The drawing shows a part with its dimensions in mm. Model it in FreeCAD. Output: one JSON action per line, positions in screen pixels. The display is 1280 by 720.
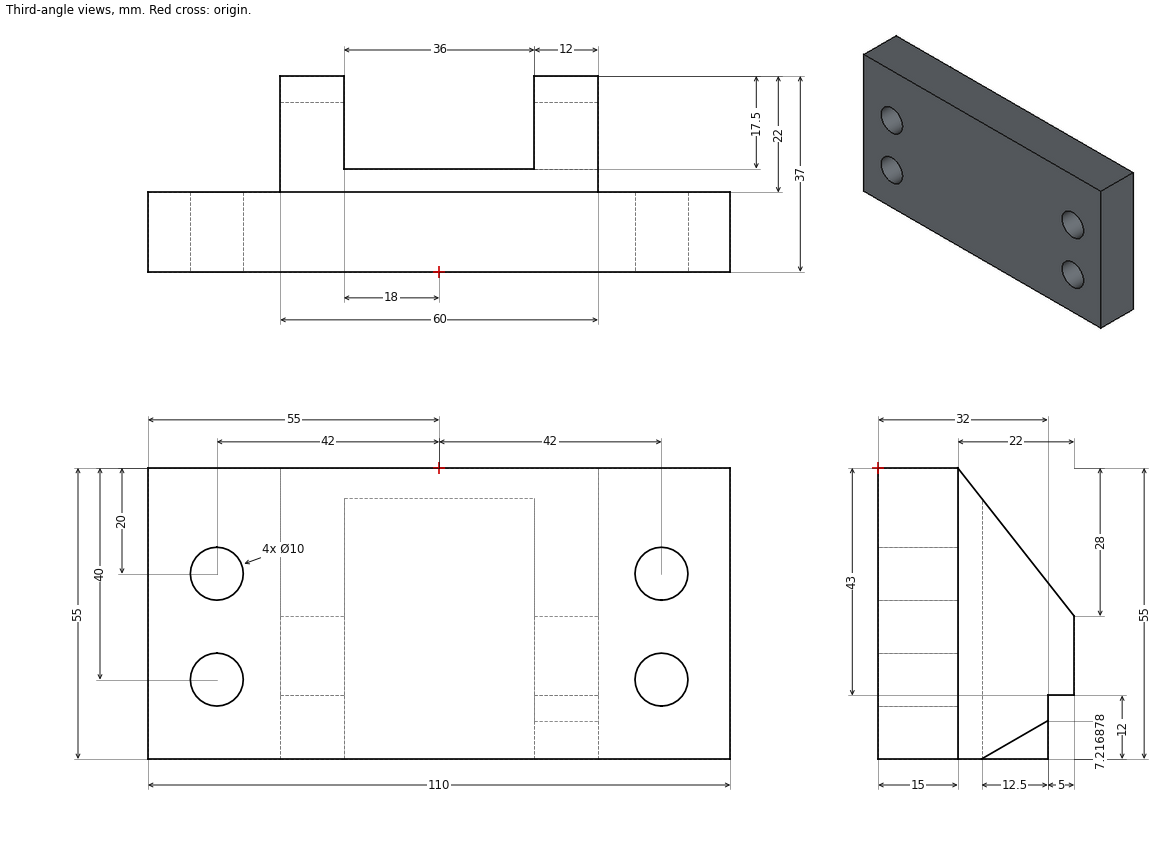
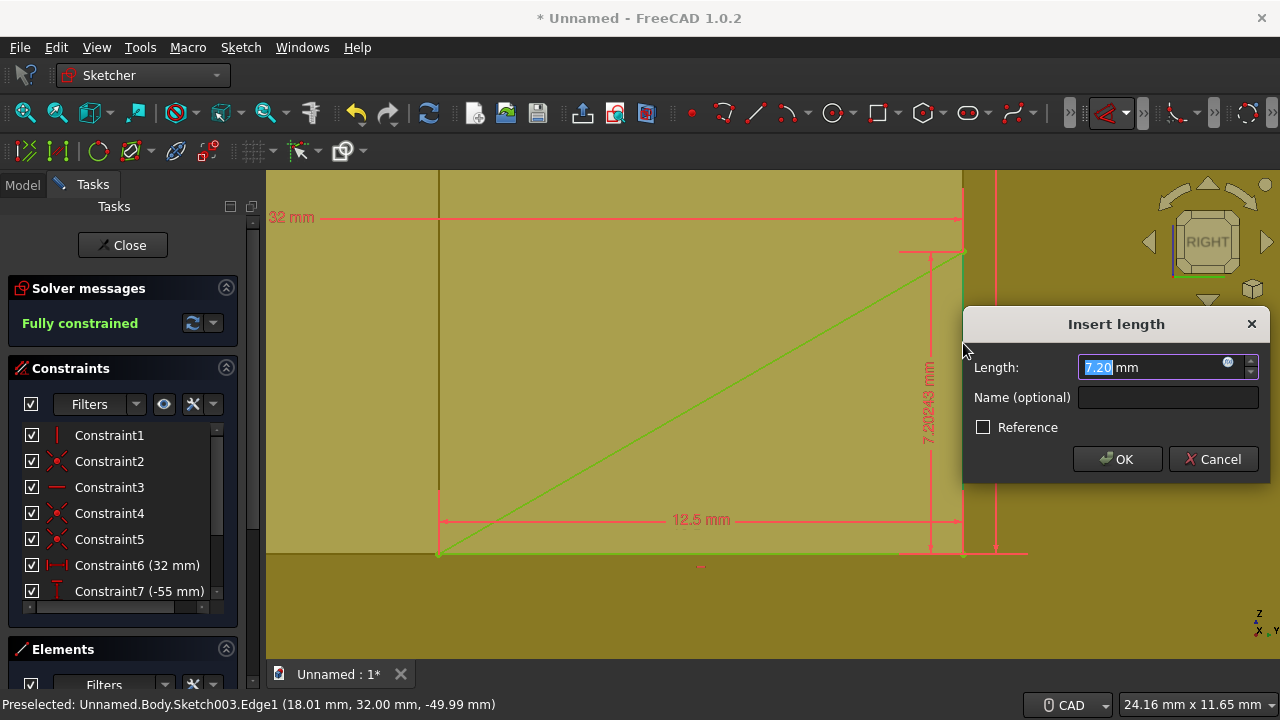
{"action": "type", "text": "7.216878"}
{"action": "key", "text": "Return"}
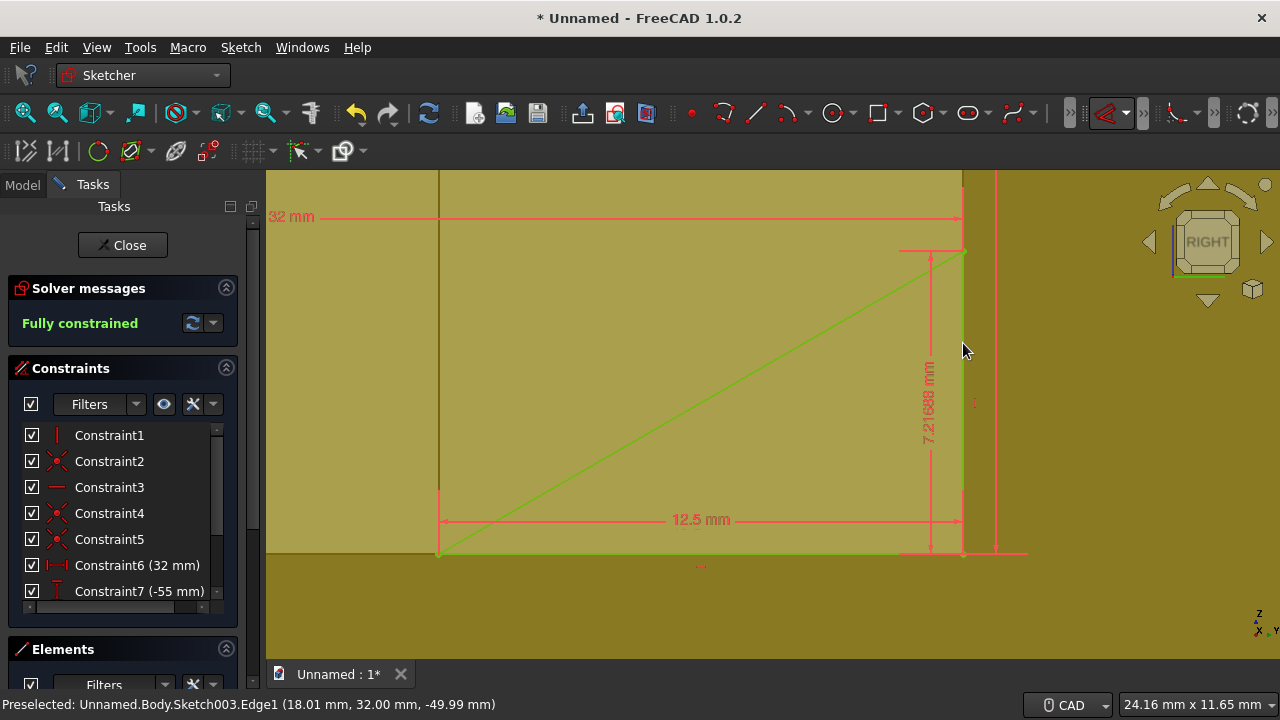
{"action": "left_click", "coordinate": [123, 245]}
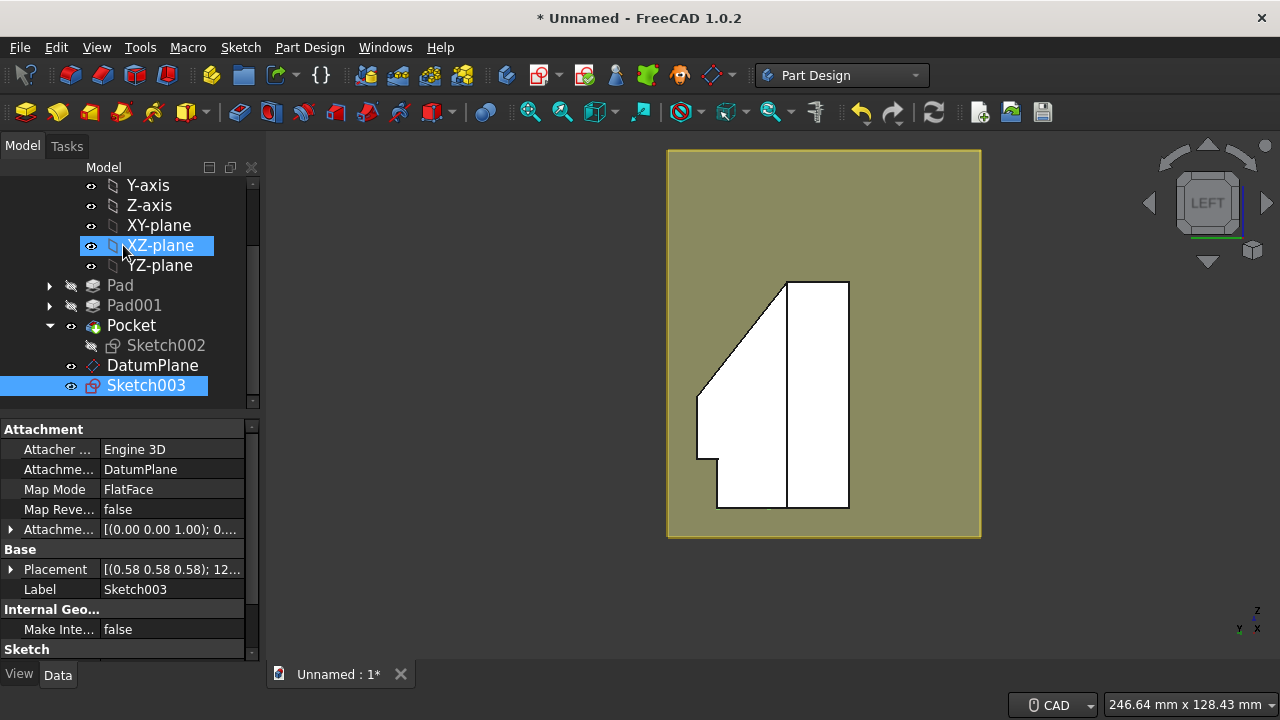
{"action": "left_click", "coordinate": [240, 112]}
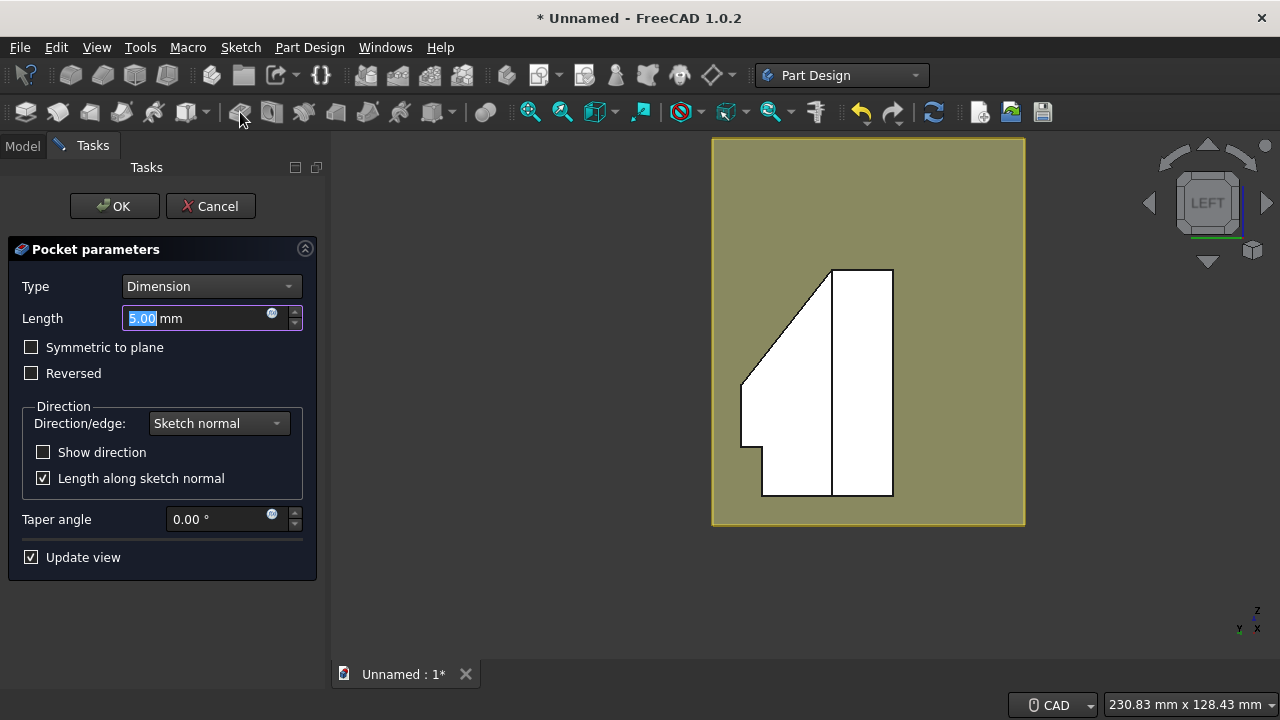
{"action": "type", "text": "12"}
{"action": "key", "text": "Tab"}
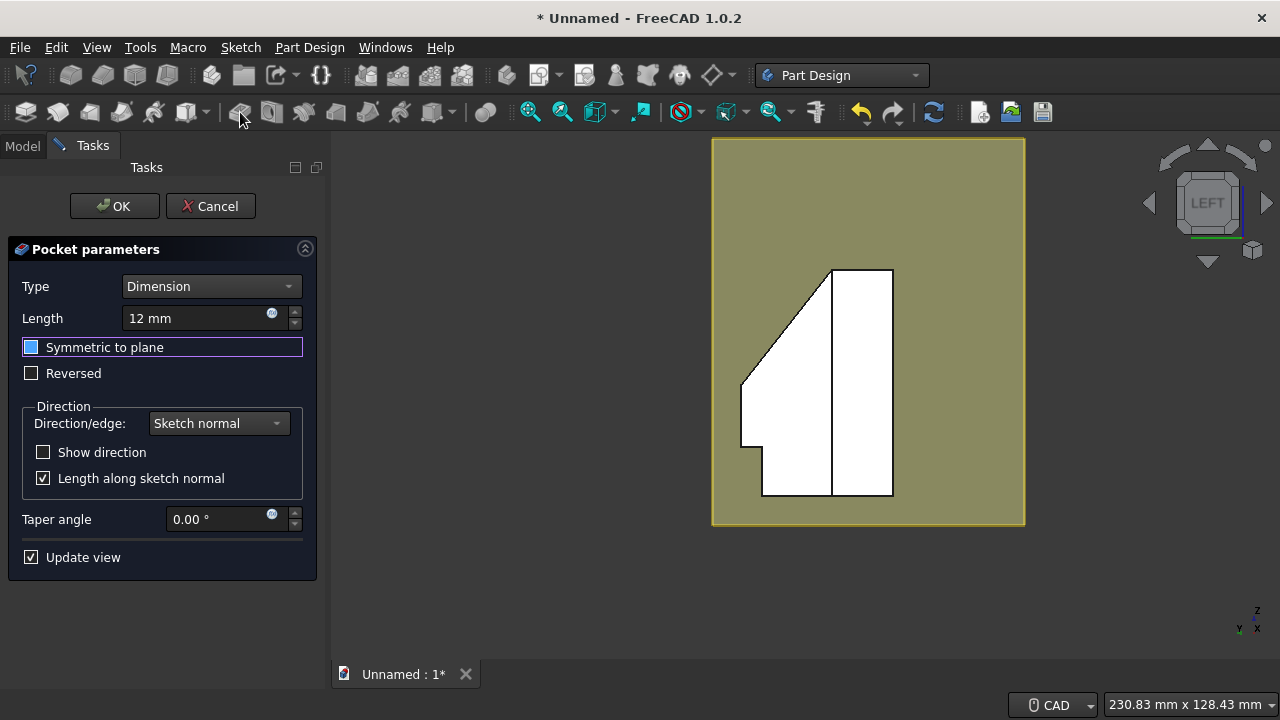
{"action": "left_click", "coordinate": [30, 373]}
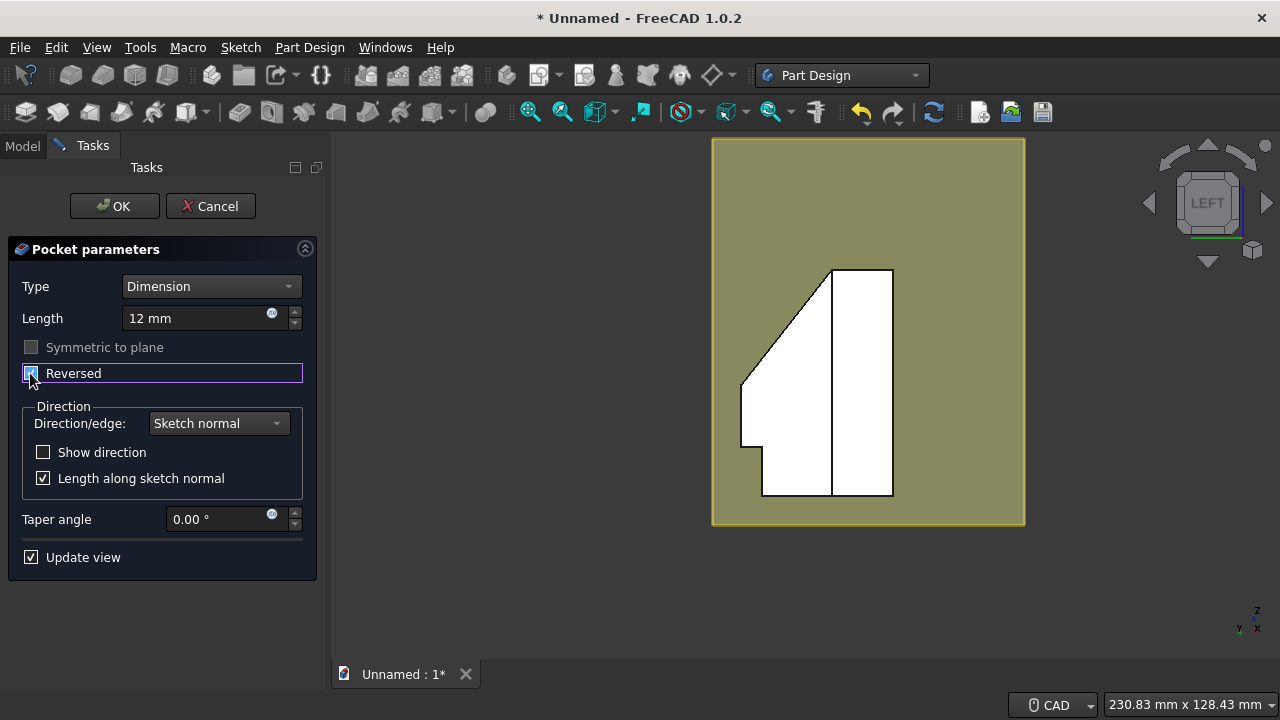
{"action": "left_click", "coordinate": [115, 206]}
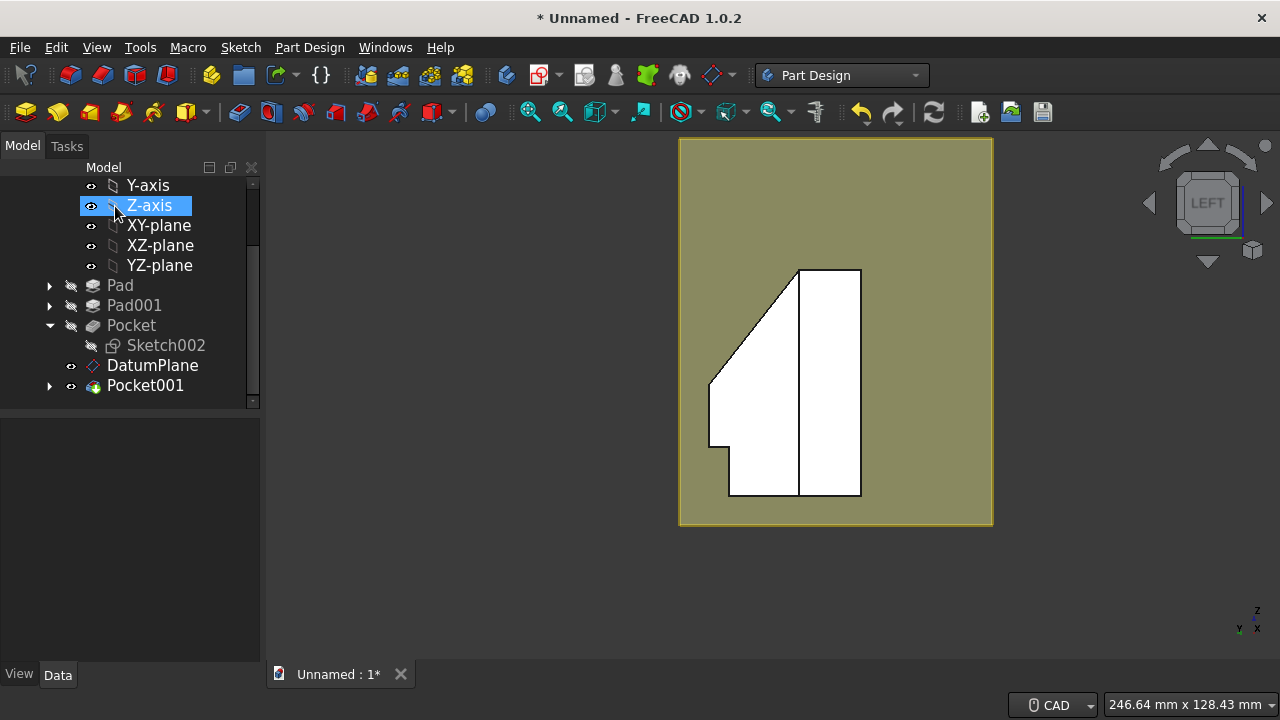
{"action": "left_click", "coordinate": [116, 366]}
{"action": "key", "text": "space"}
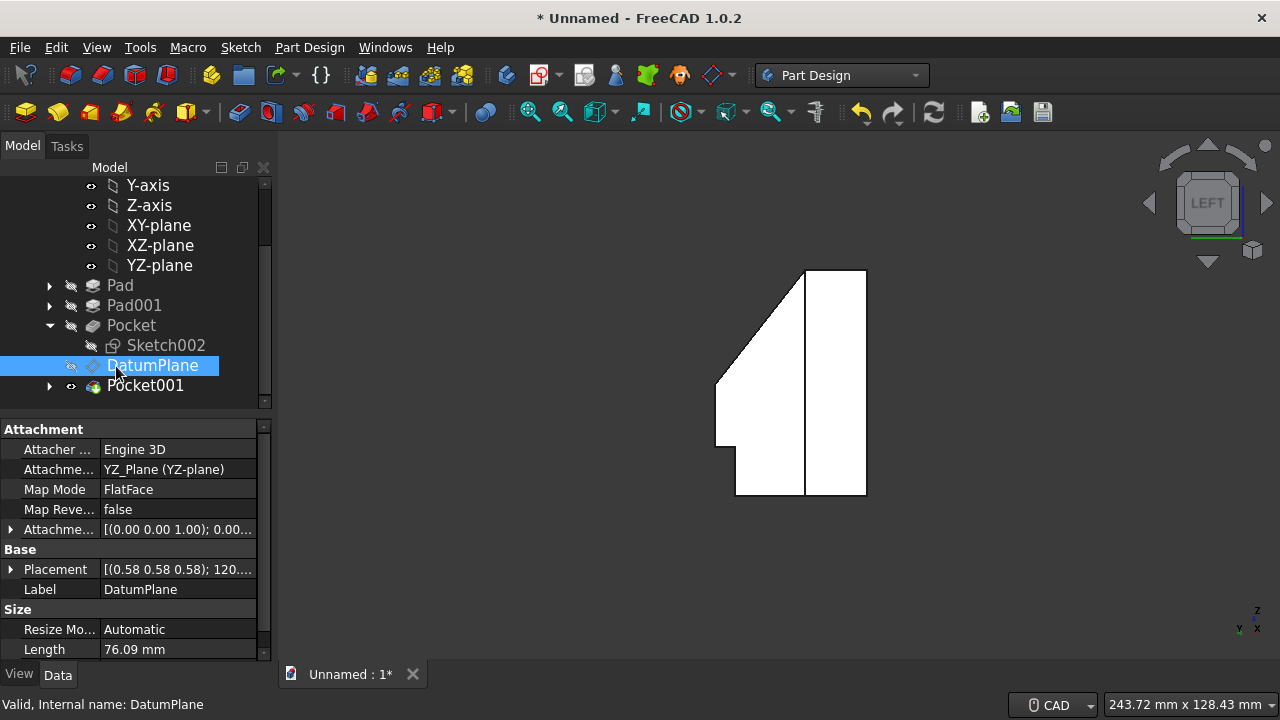
{"action": "key", "text": "0"}